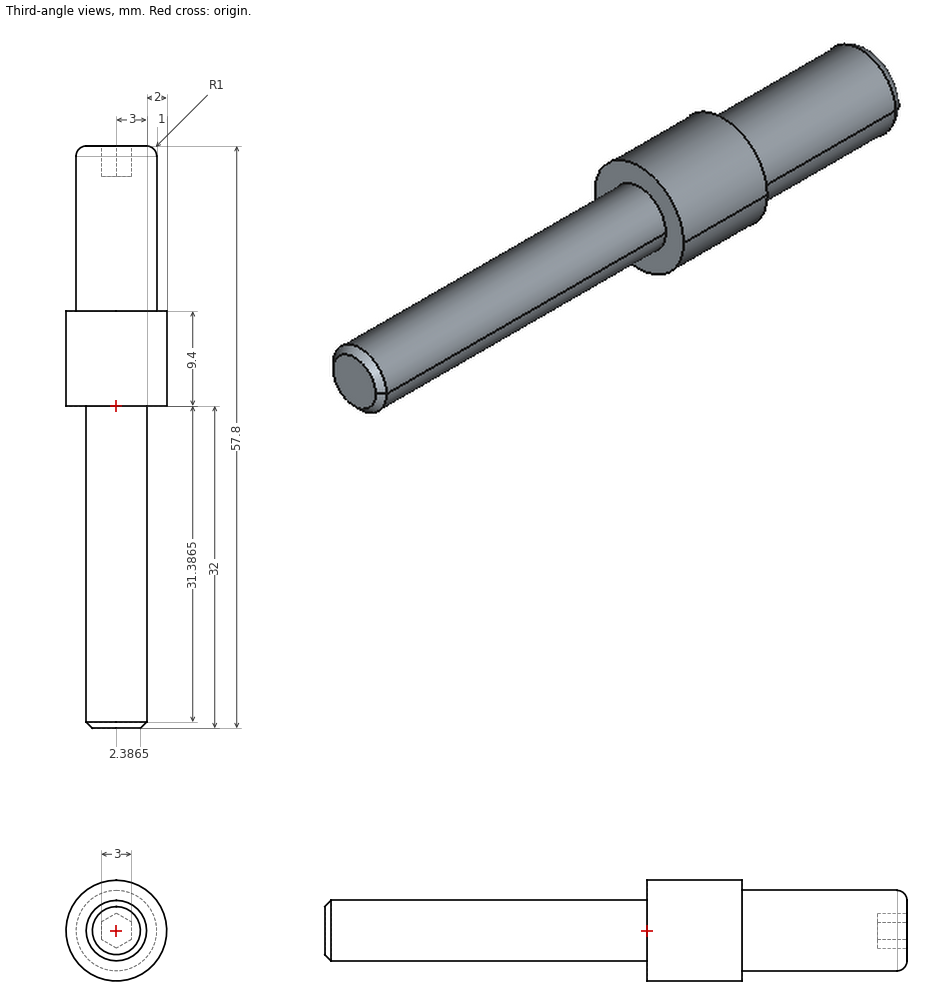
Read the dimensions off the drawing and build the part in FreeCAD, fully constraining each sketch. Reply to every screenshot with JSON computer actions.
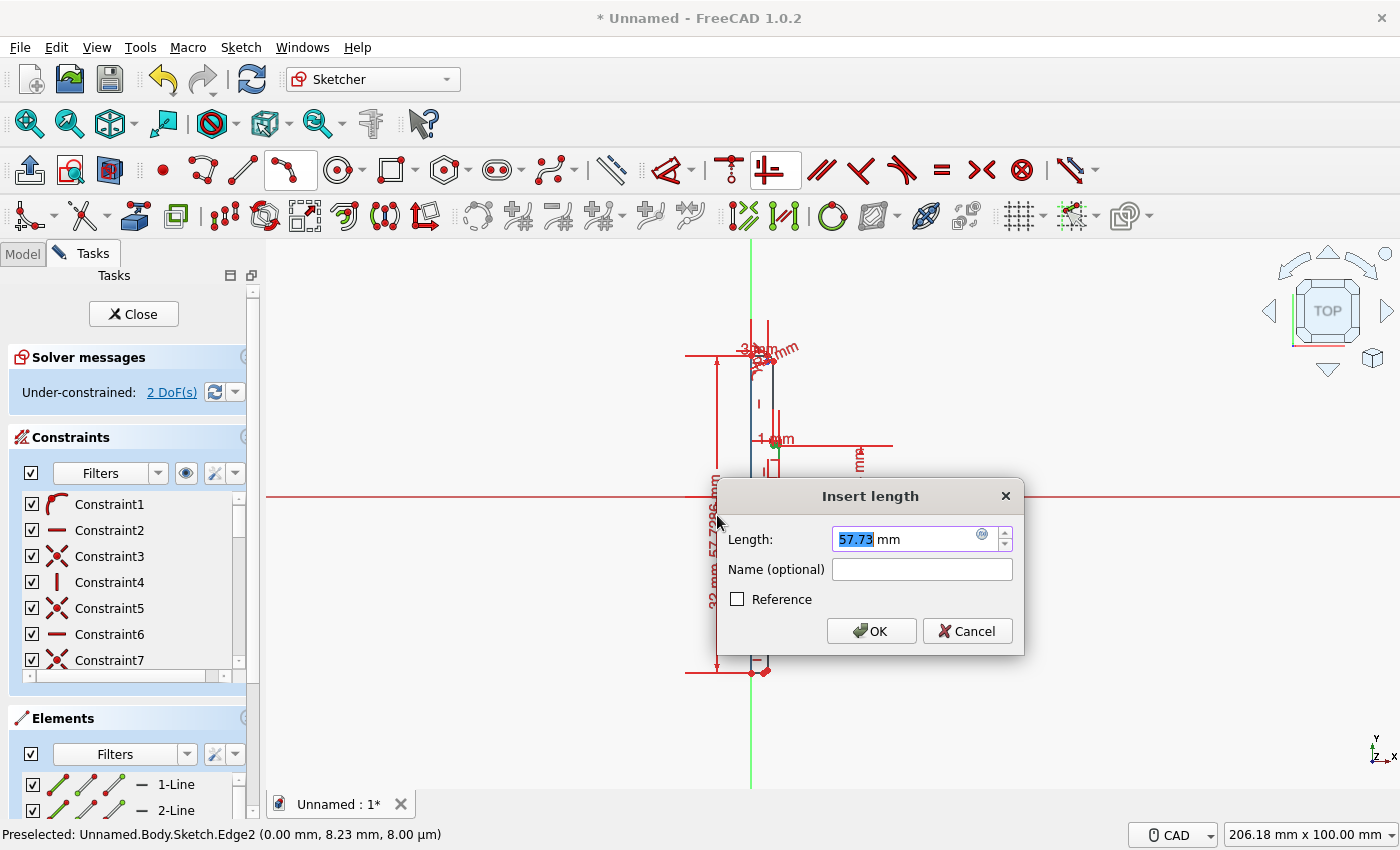
{"action": "type", "text": "57.8"}
{"action": "key", "text": "Return"}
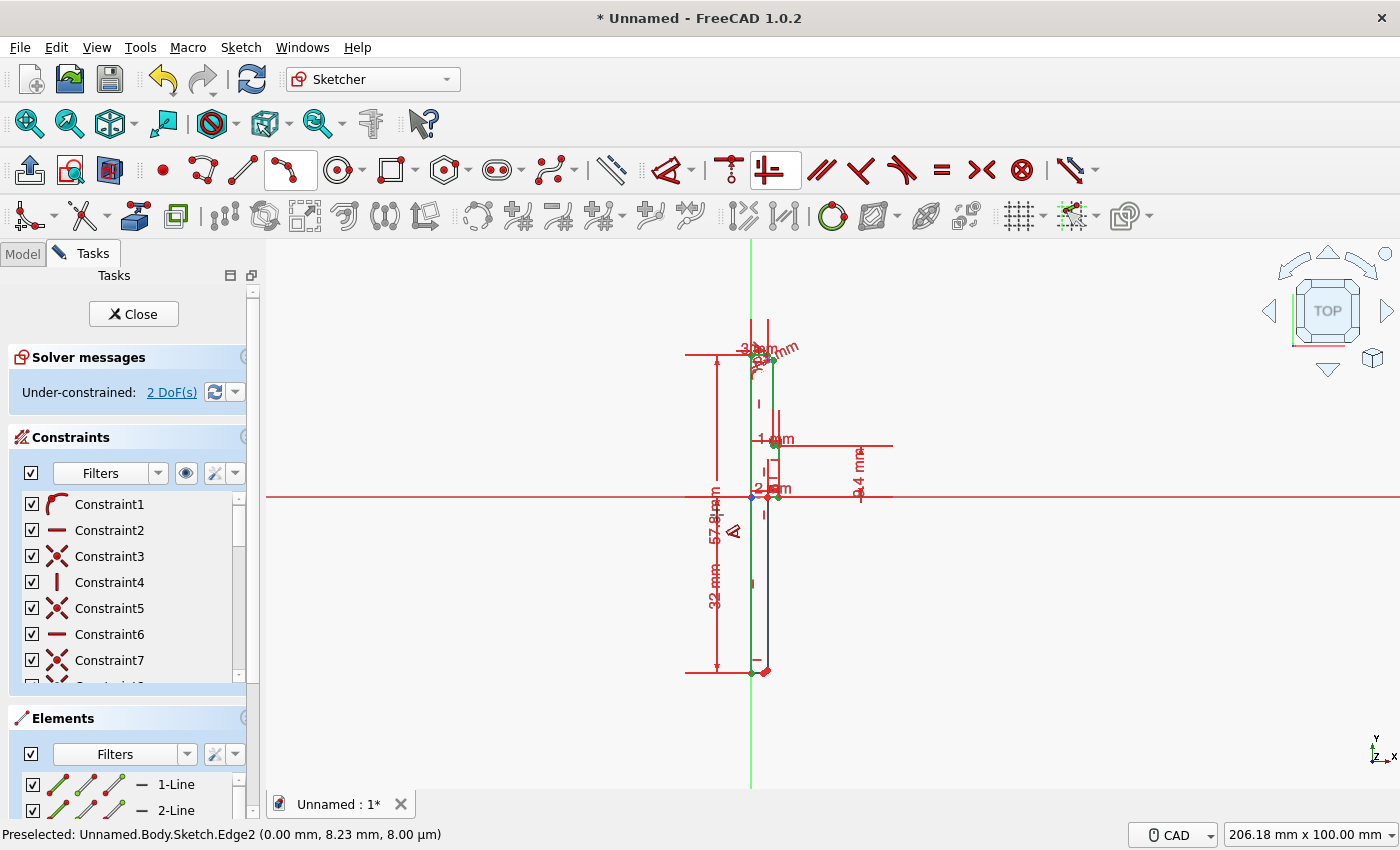
{"action": "scroll", "coordinate": [757, 673], "scroll_direction": "up", "scroll_amount": 6}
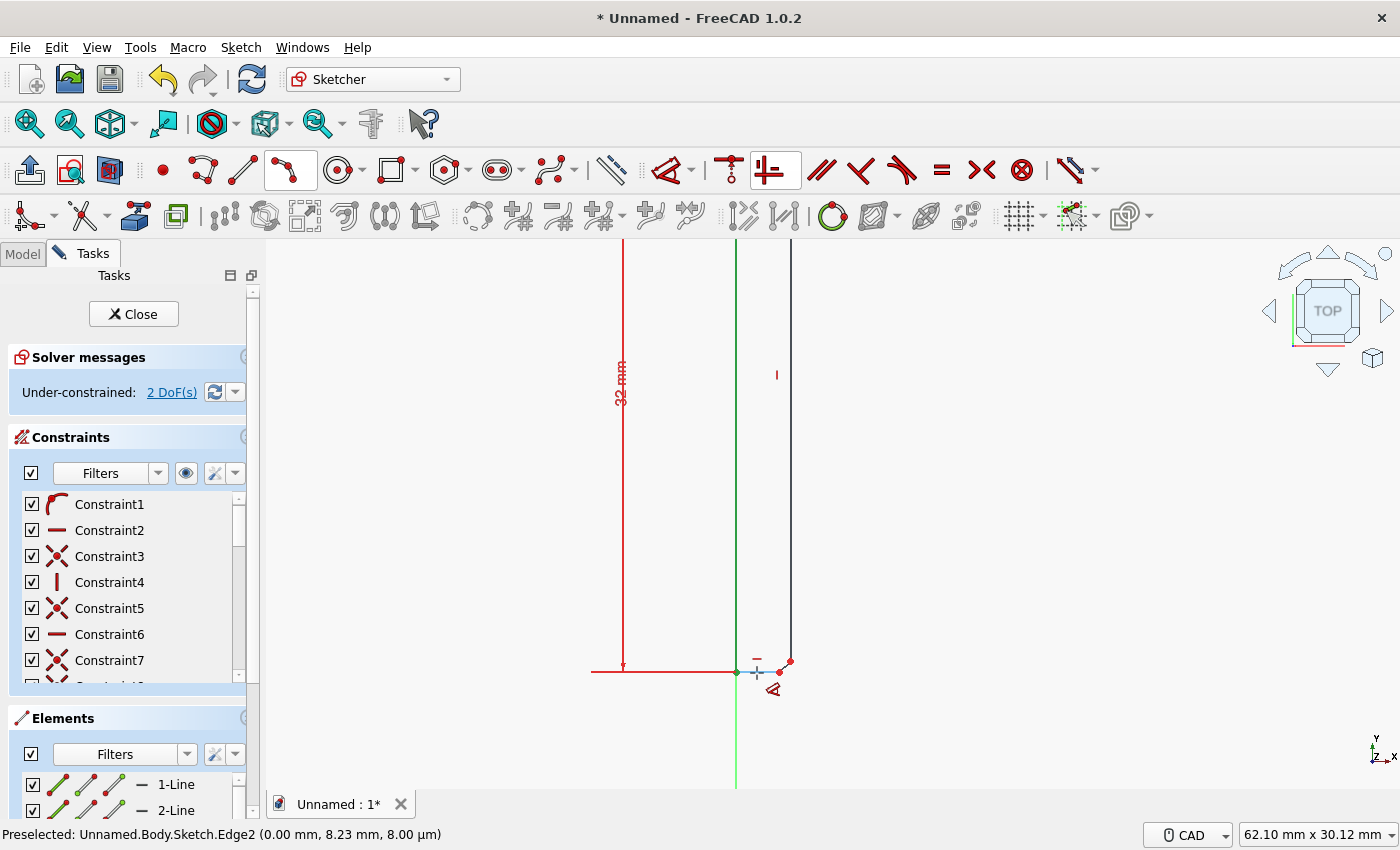
{"action": "left_click", "coordinate": [758, 672]}
{"action": "left_click", "coordinate": [758, 706]}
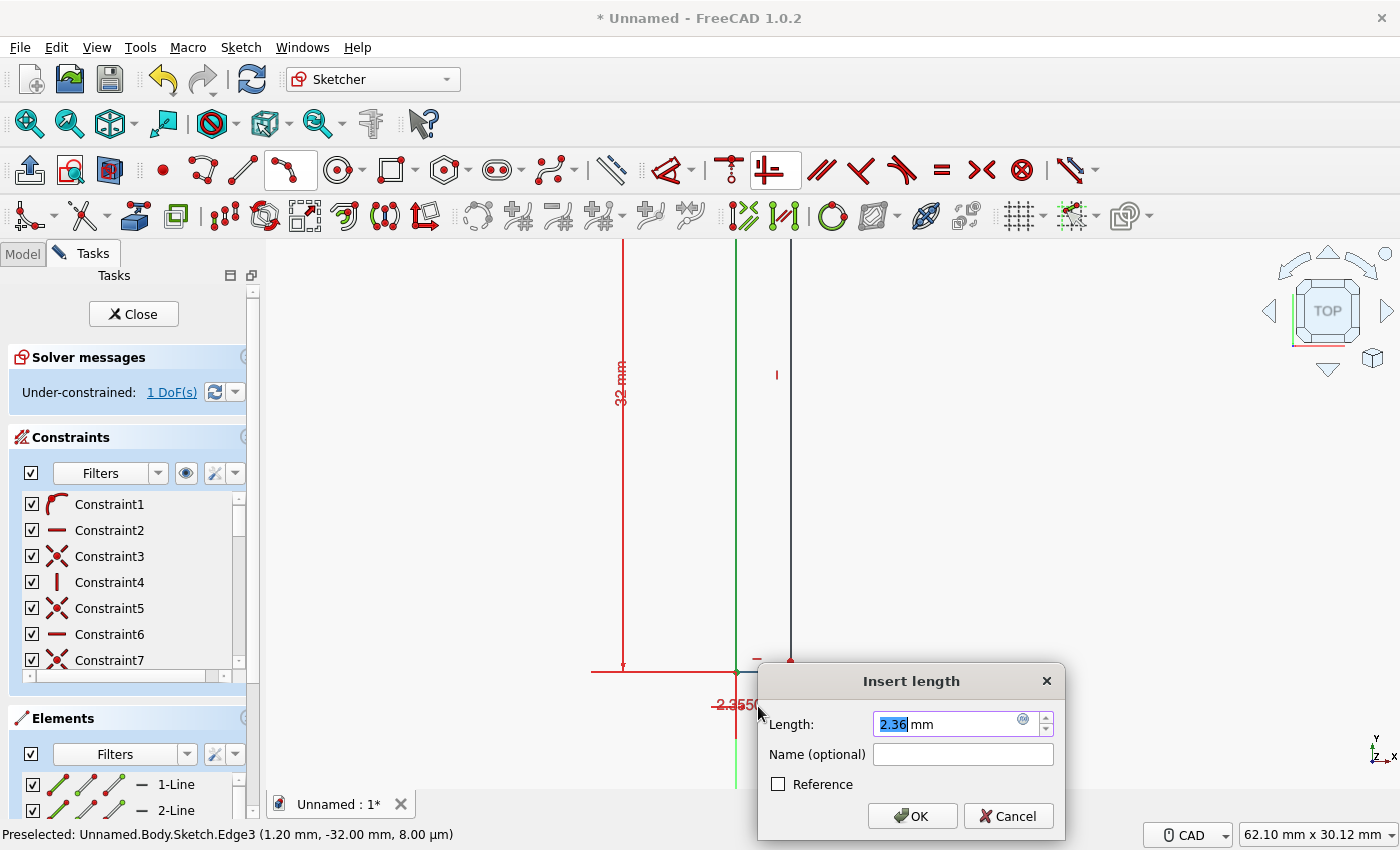
{"action": "type", "text": "2.3865"}
{"action": "key", "text": "Return"}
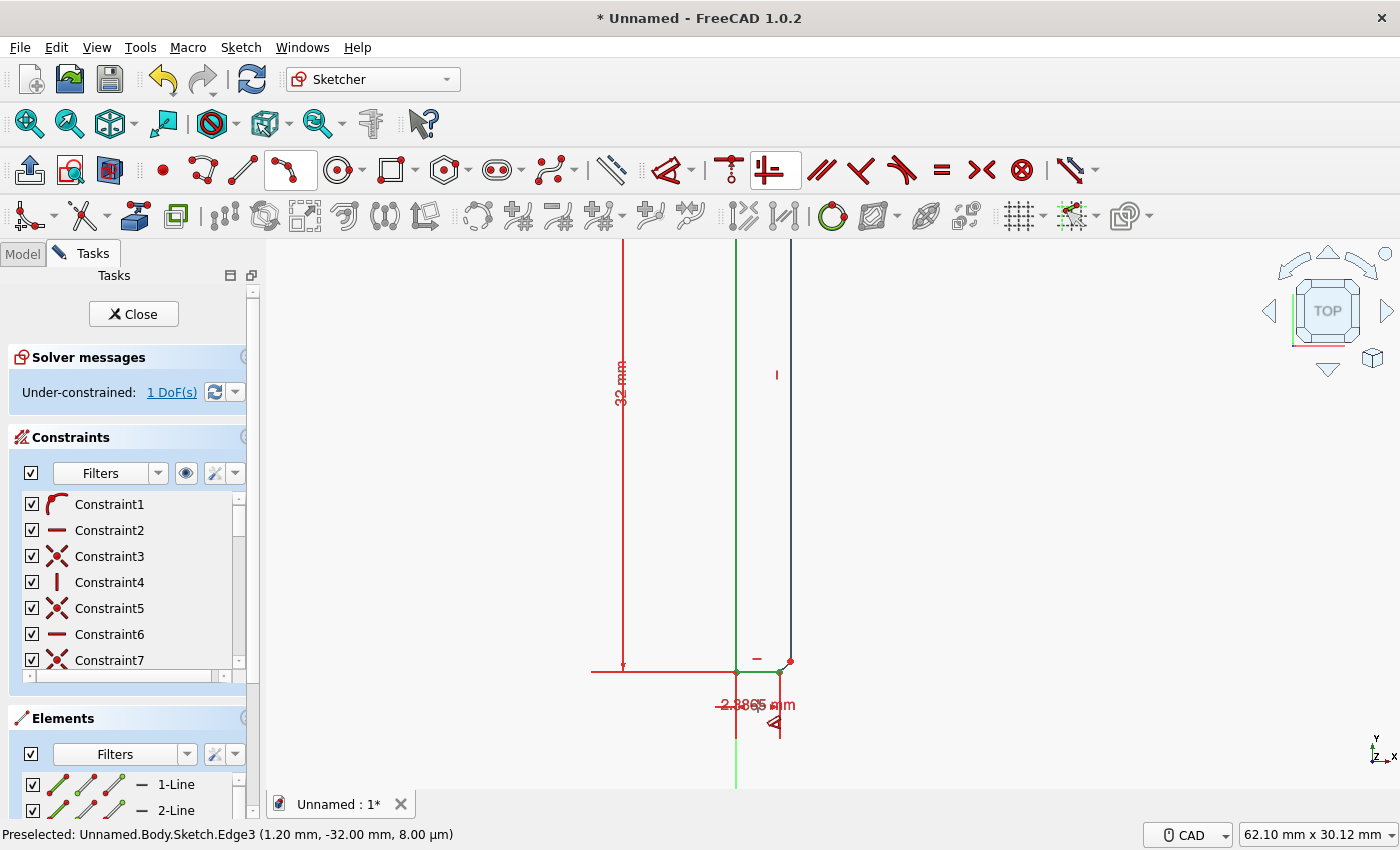
{"action": "left_click", "coordinate": [791, 490]}
{"action": "left_click", "coordinate": [825, 464]}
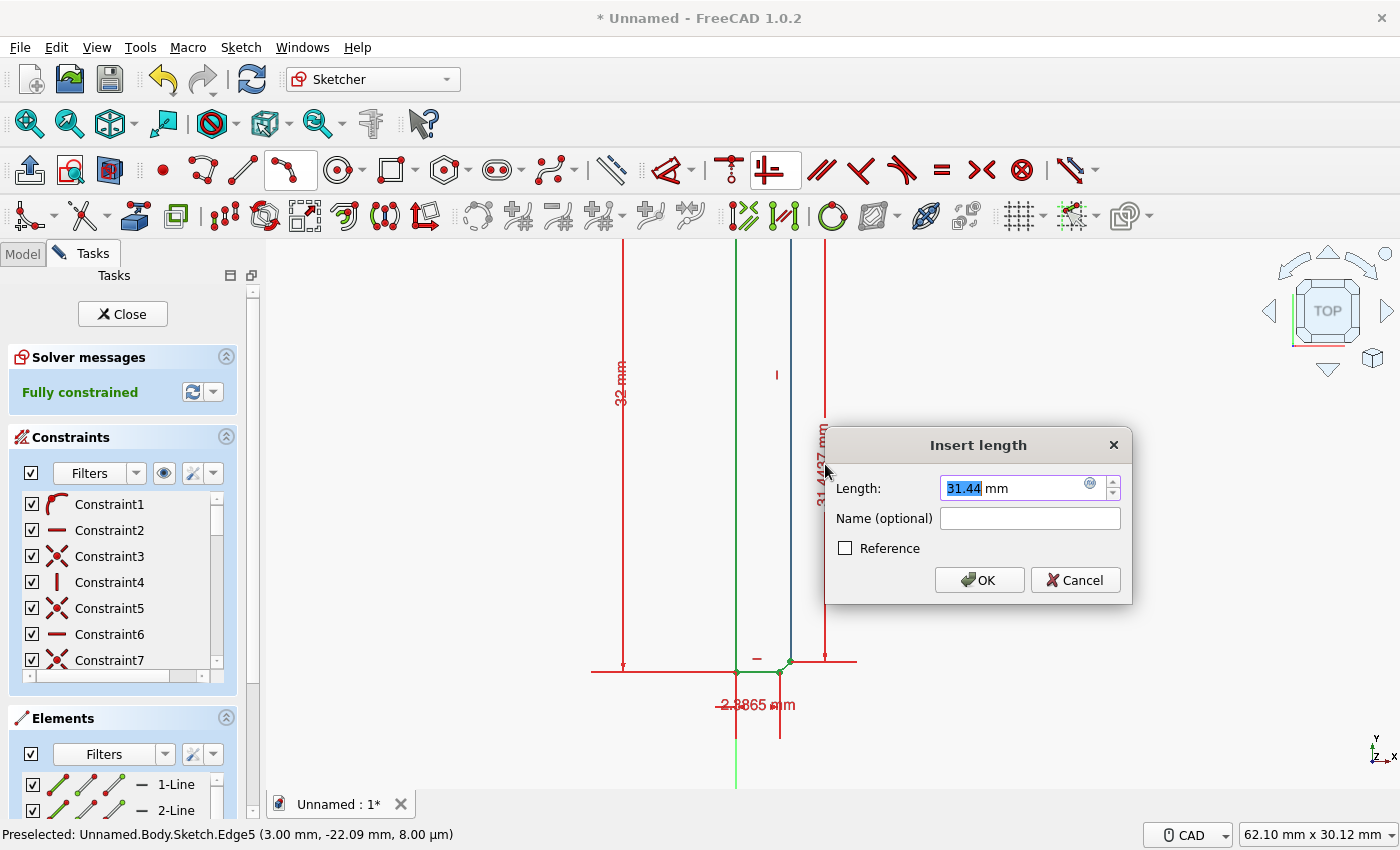
{"action": "type", "text": "31.3865"}
{"action": "key", "text": "Return"}
{"action": "key", "text": "Escape"}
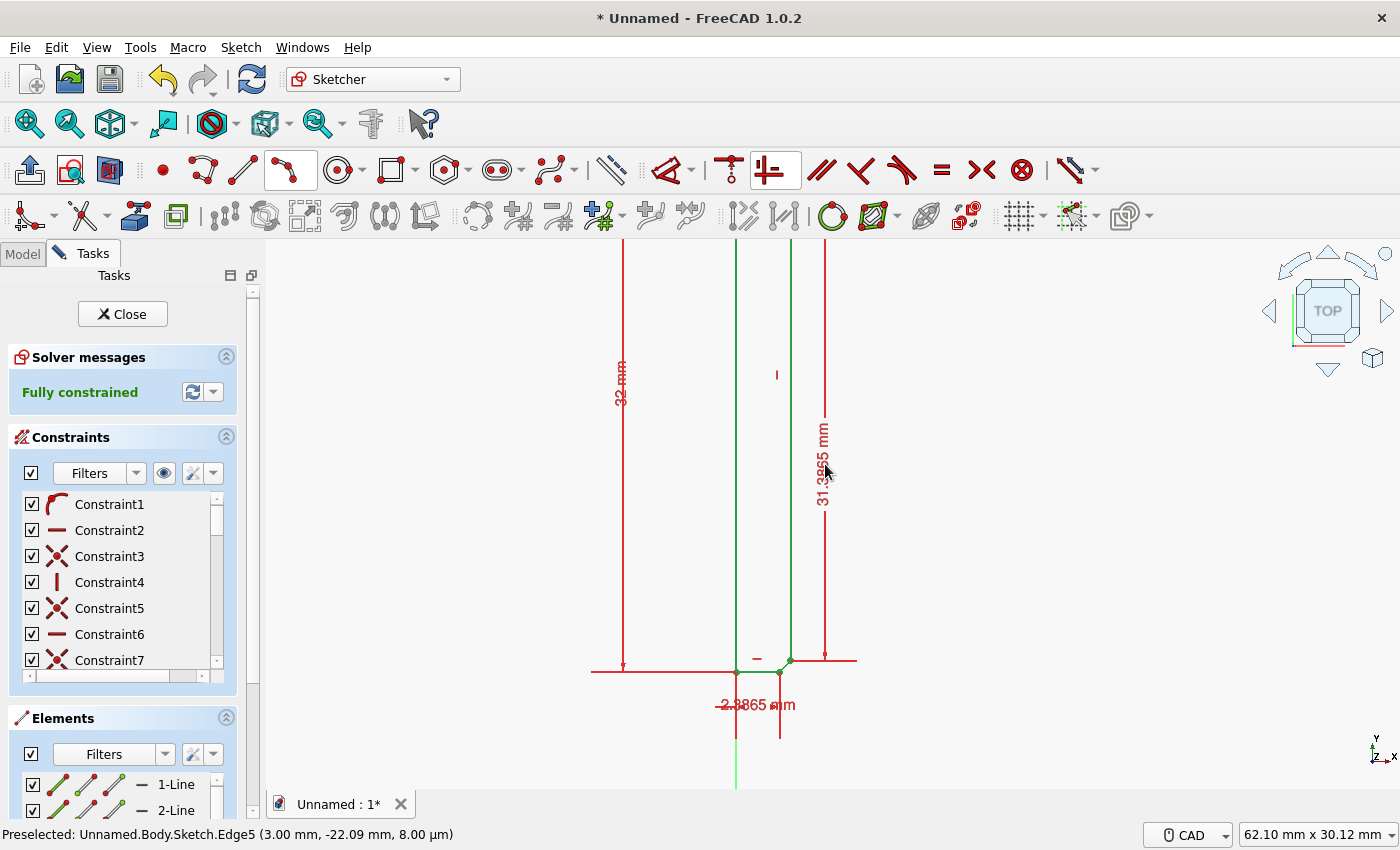
{"action": "left_click", "coordinate": [123, 314]}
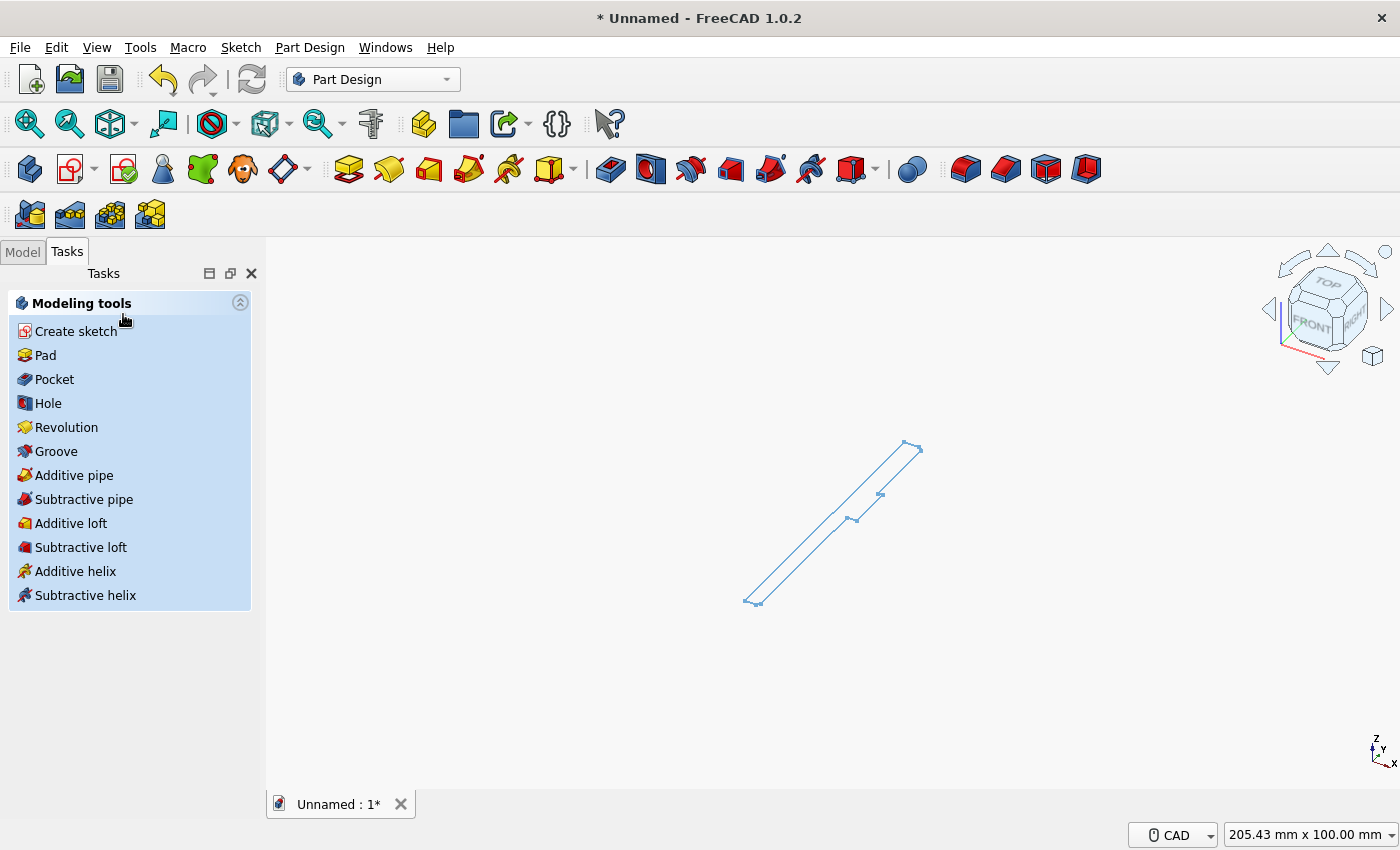
{"action": "left_click", "coordinate": [390, 170]}